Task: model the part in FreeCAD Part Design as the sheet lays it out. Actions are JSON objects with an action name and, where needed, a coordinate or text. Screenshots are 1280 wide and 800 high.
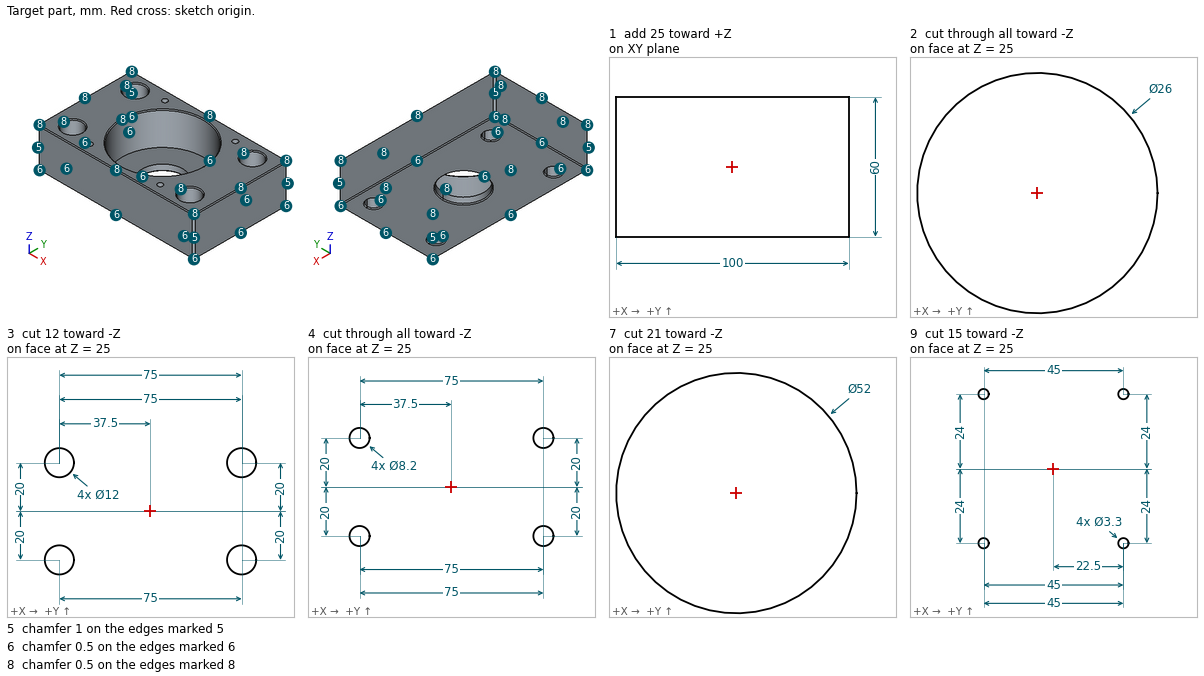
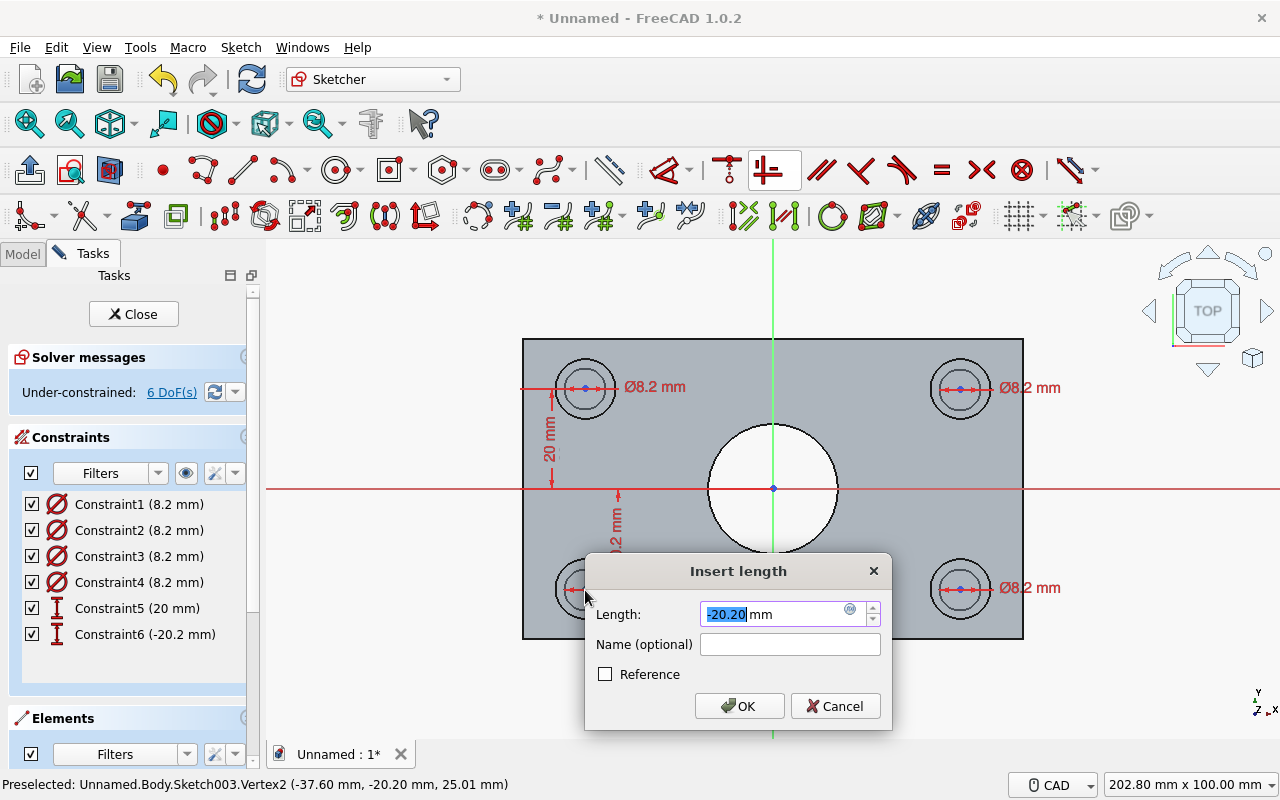
{"action": "type", "text": "-20"}
{"action": "key", "text": "Return"}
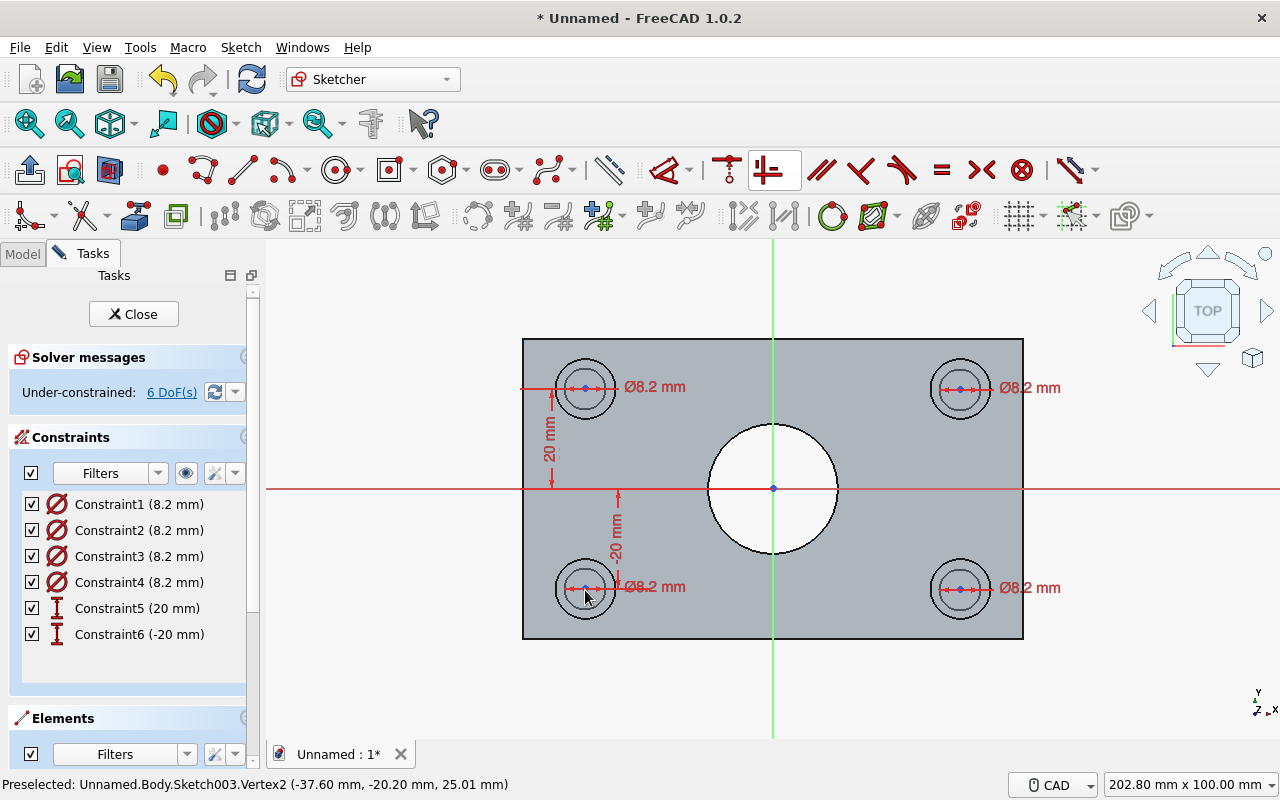
{"action": "left_click", "coordinate": [960, 390]}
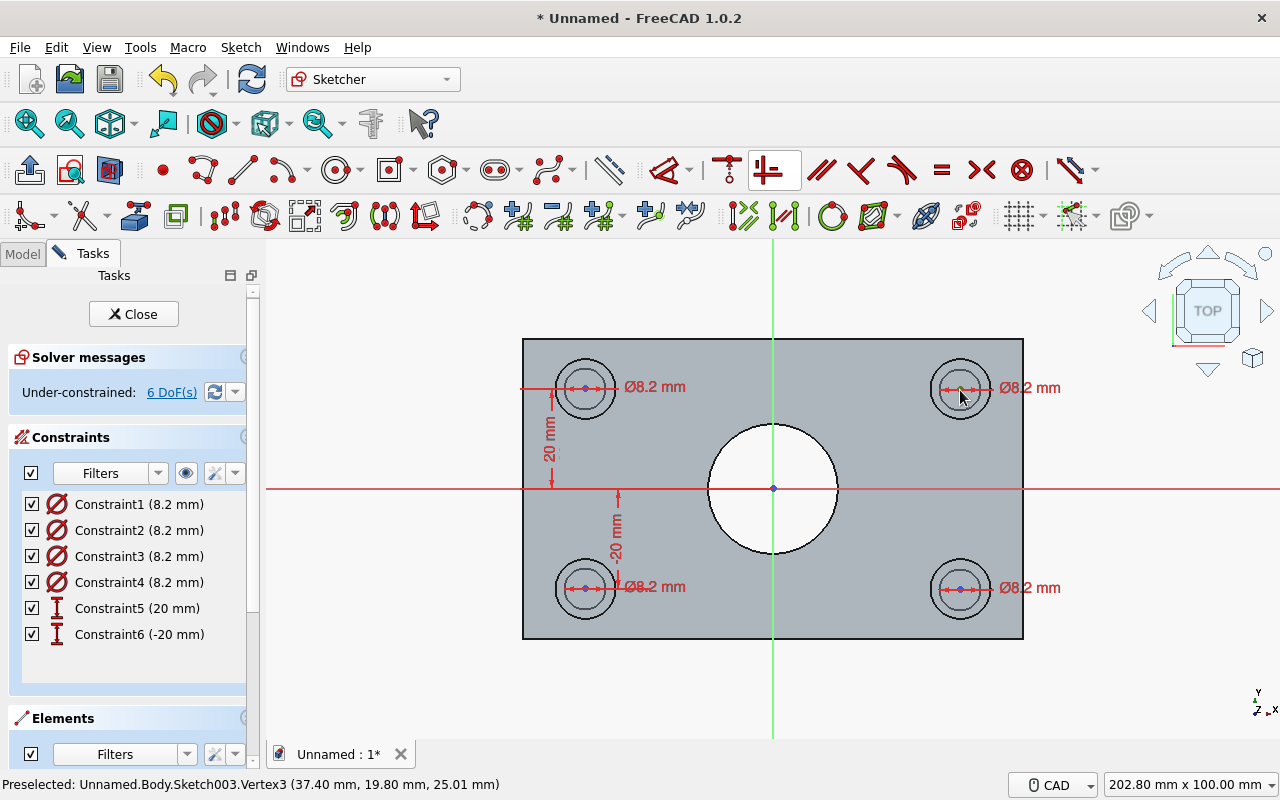
{"action": "key", "text": "i"}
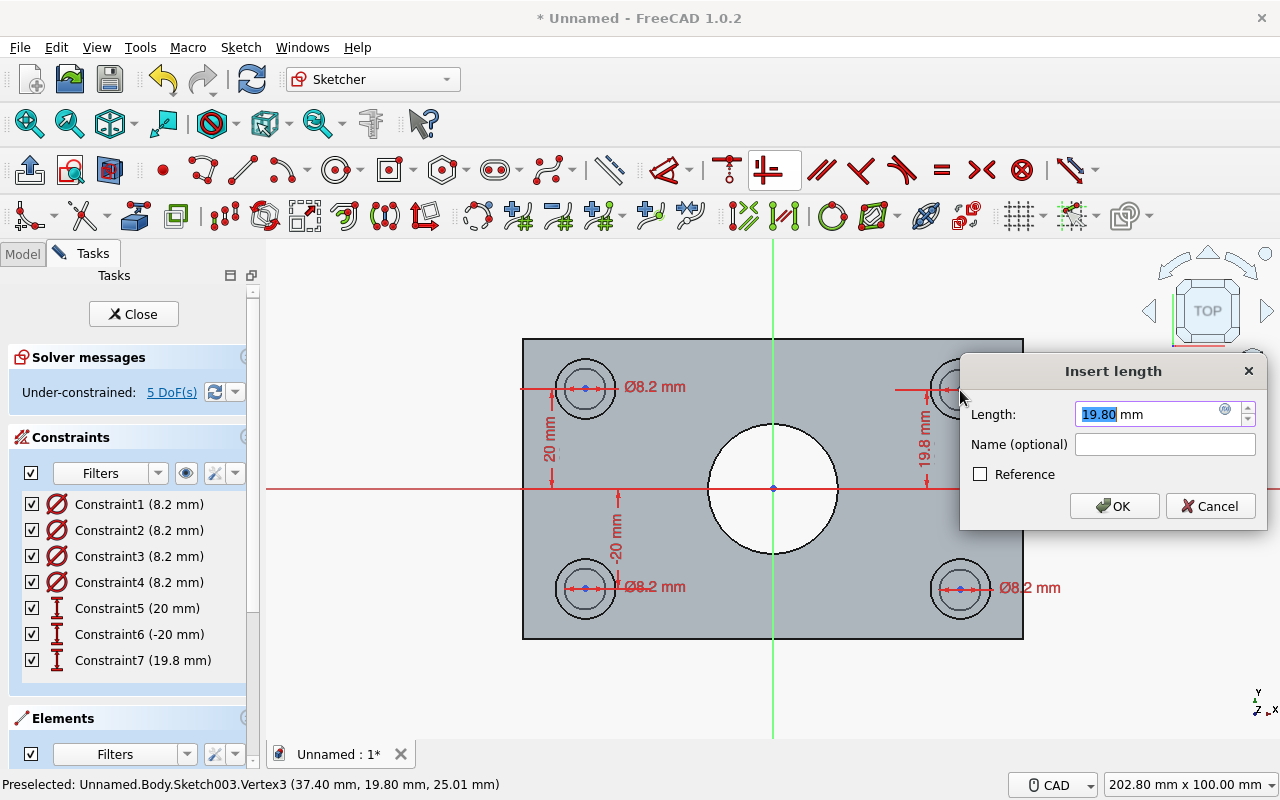
{"action": "type", "text": "20"}
{"action": "key", "text": "Return"}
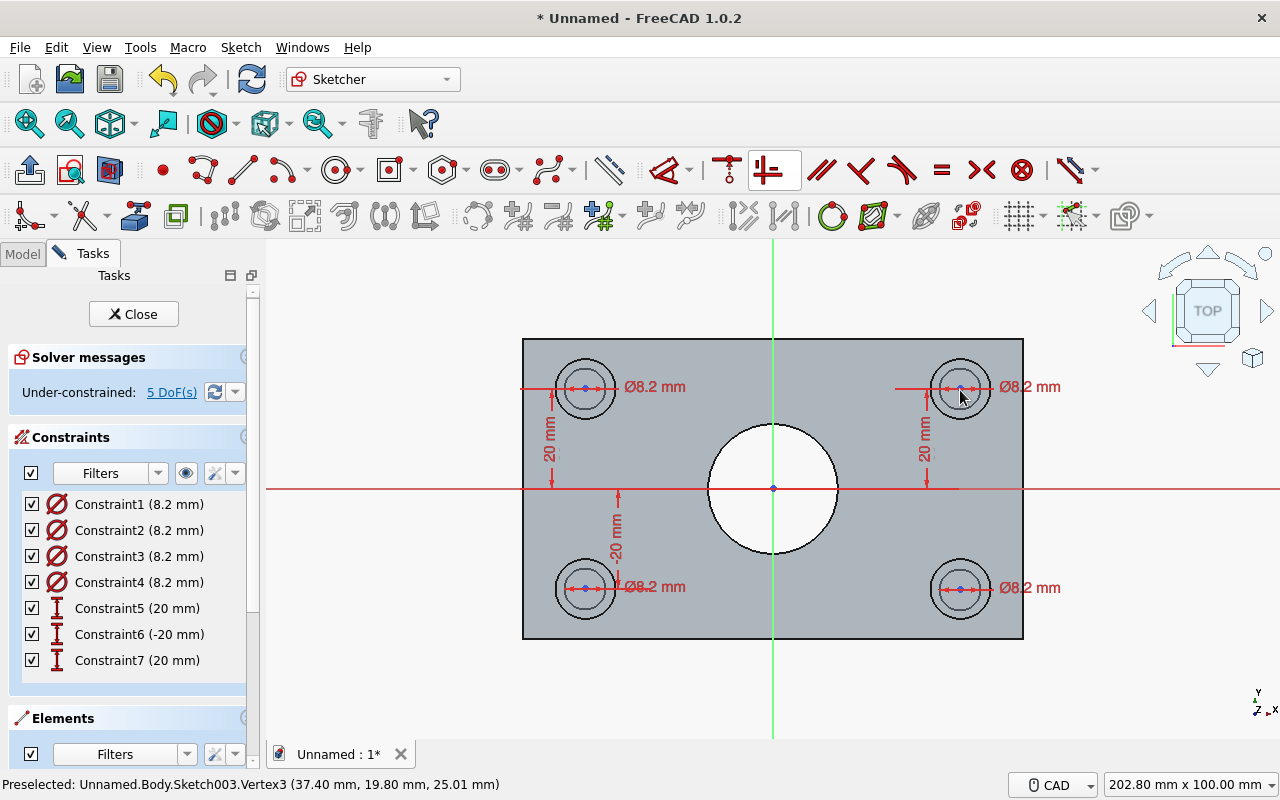
{"action": "left_click", "coordinate": [960, 590]}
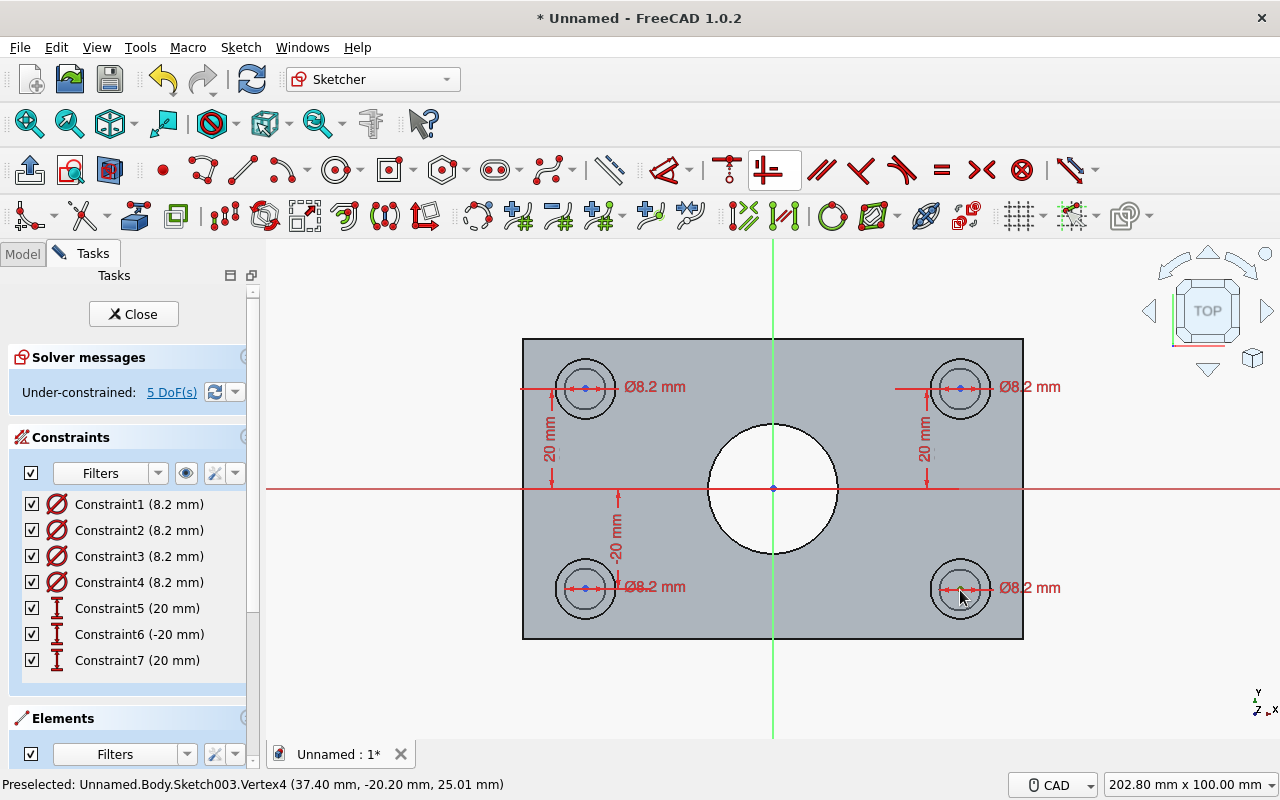
{"action": "key", "text": "i"}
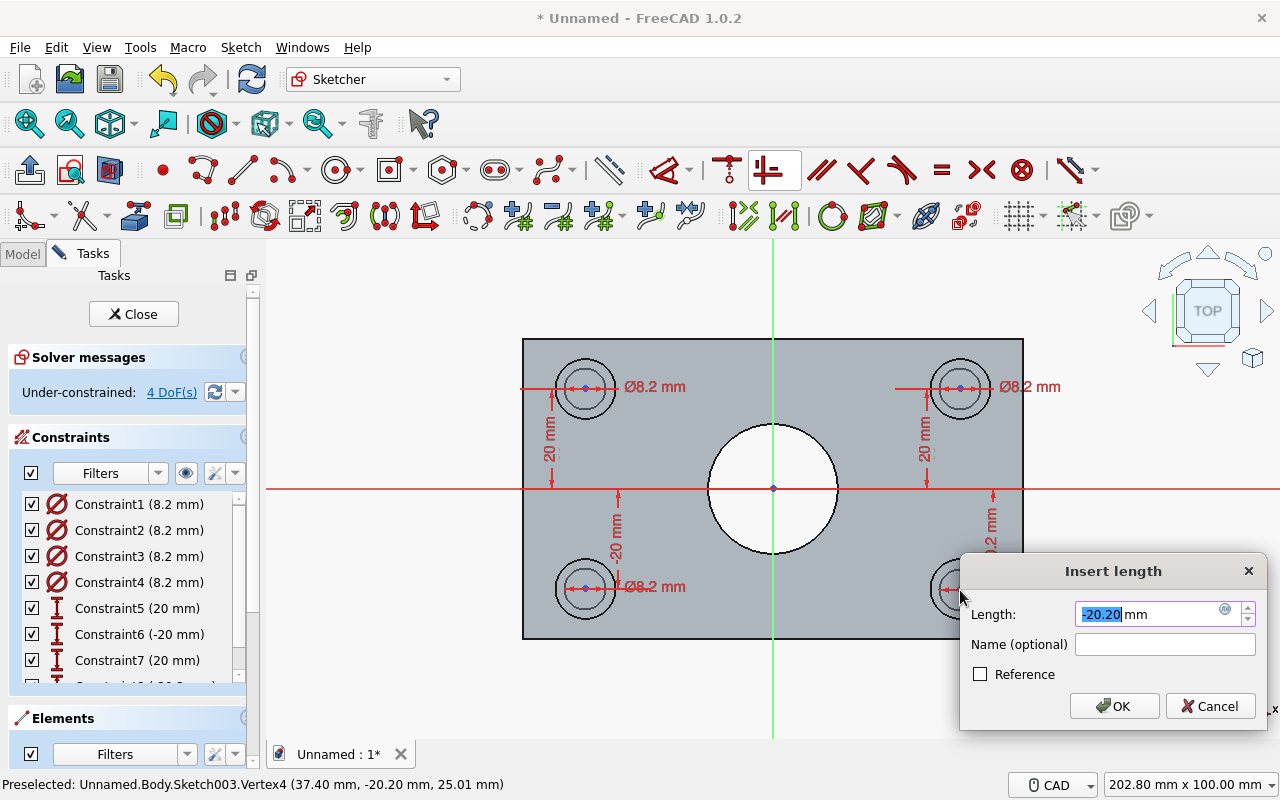
{"action": "type", "text": "-20"}
{"action": "key", "text": "Return"}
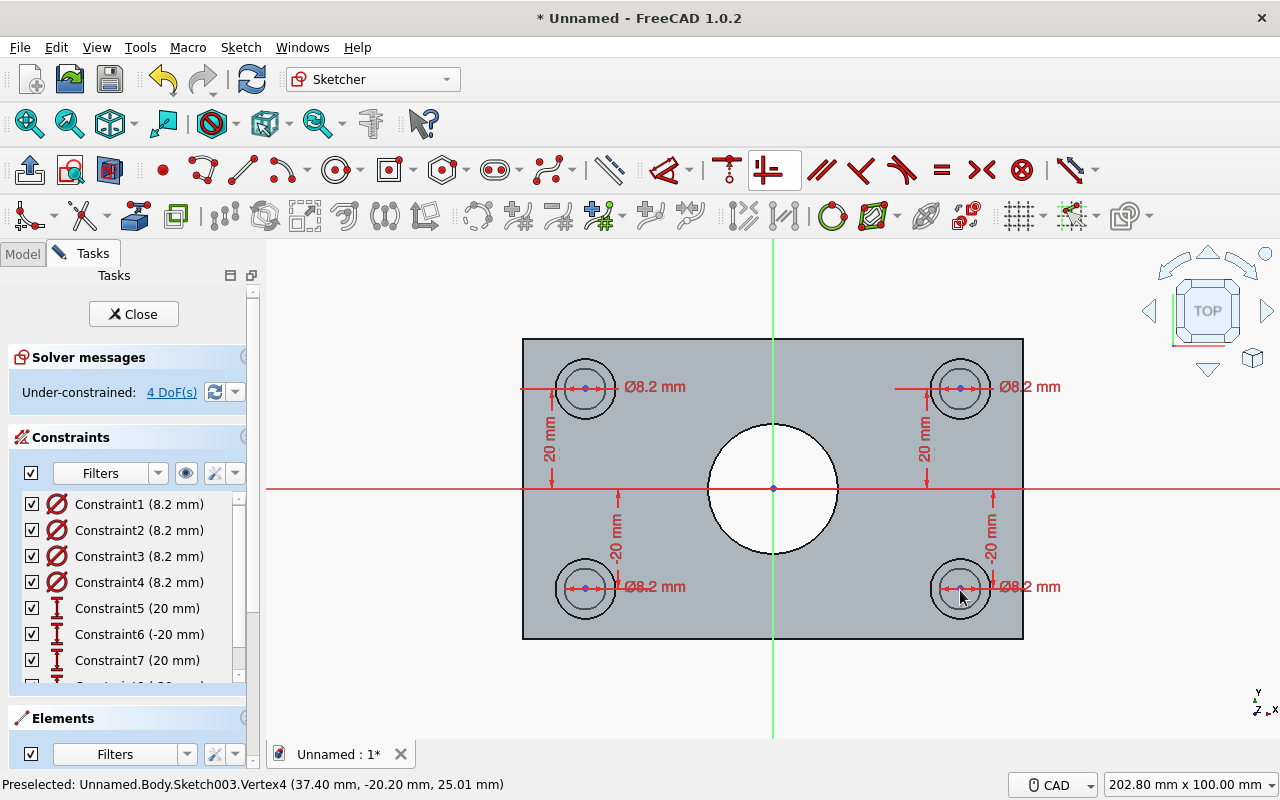
{"action": "left_click", "coordinate": [585, 389]}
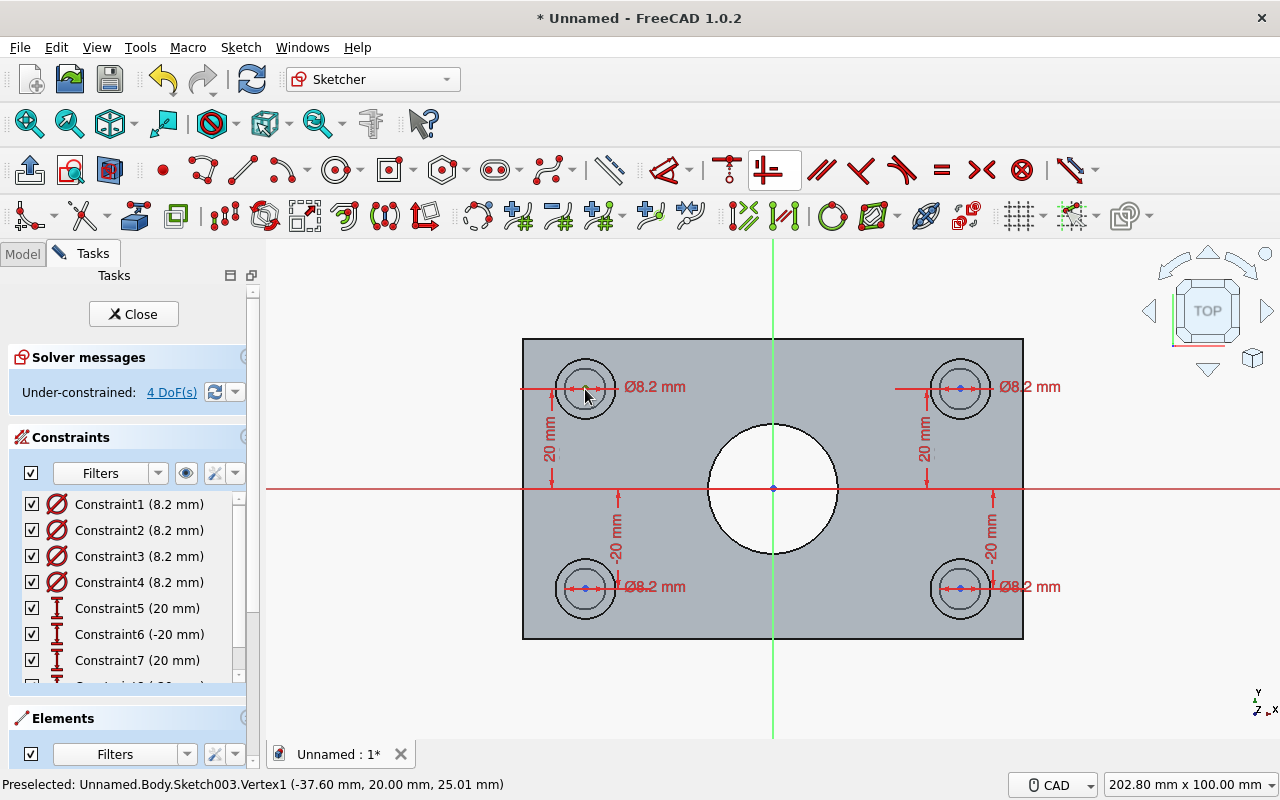
{"action": "left_click", "coordinate": [960, 389]}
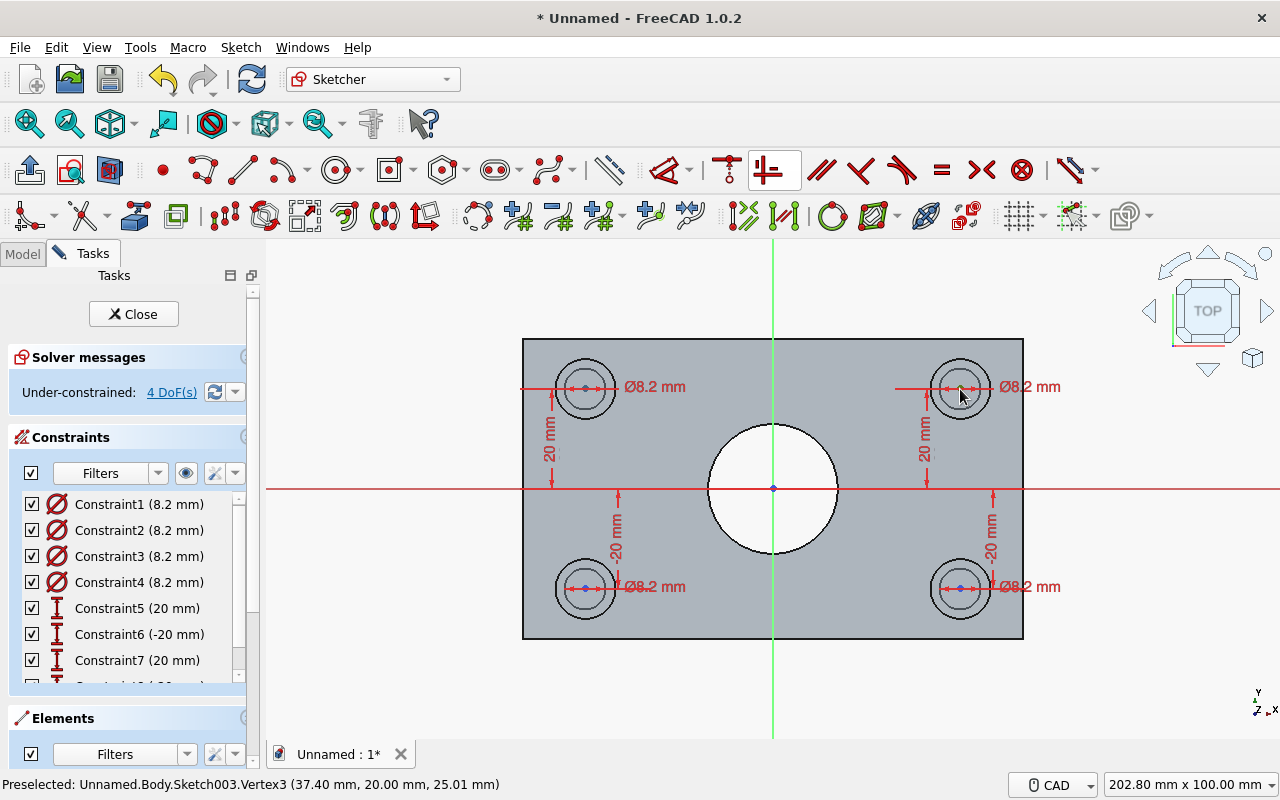
{"action": "key", "text": "l"}